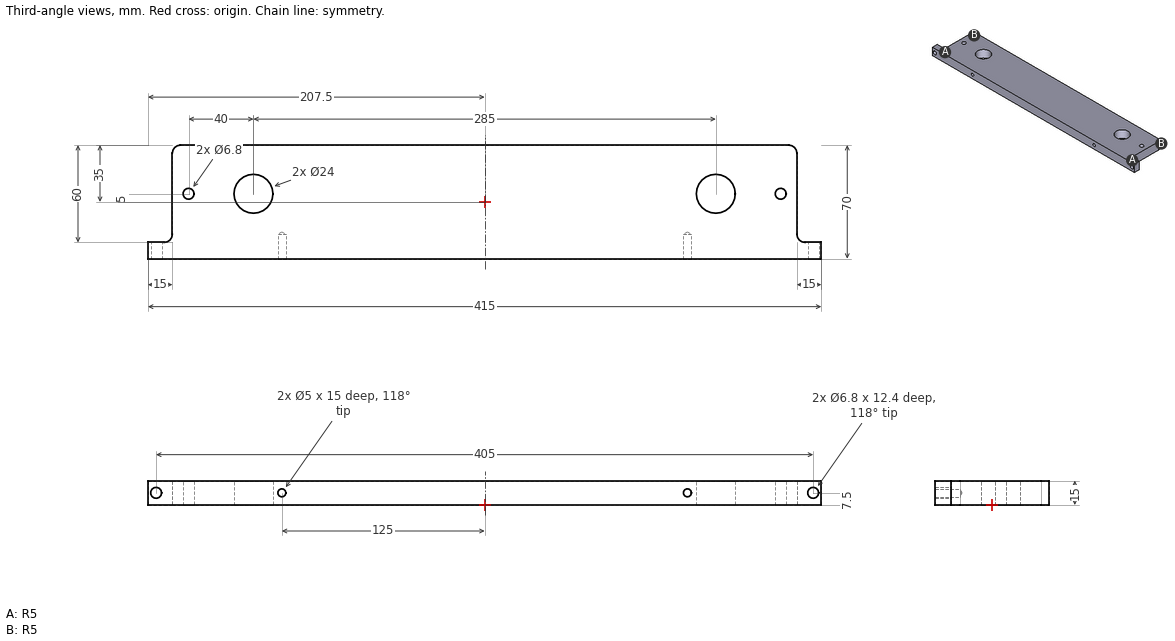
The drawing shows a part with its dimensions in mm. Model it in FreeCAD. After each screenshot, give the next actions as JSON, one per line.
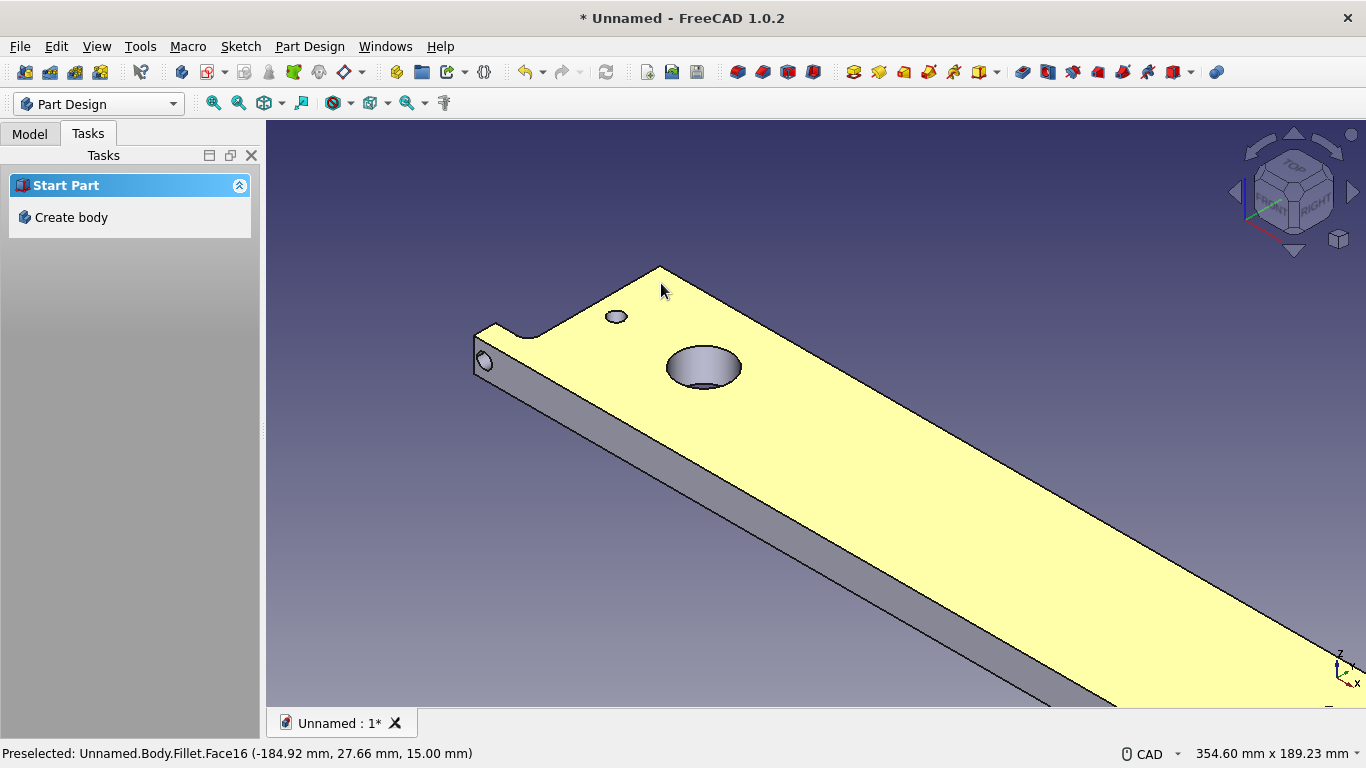
{"action": "key", "text": "v f"}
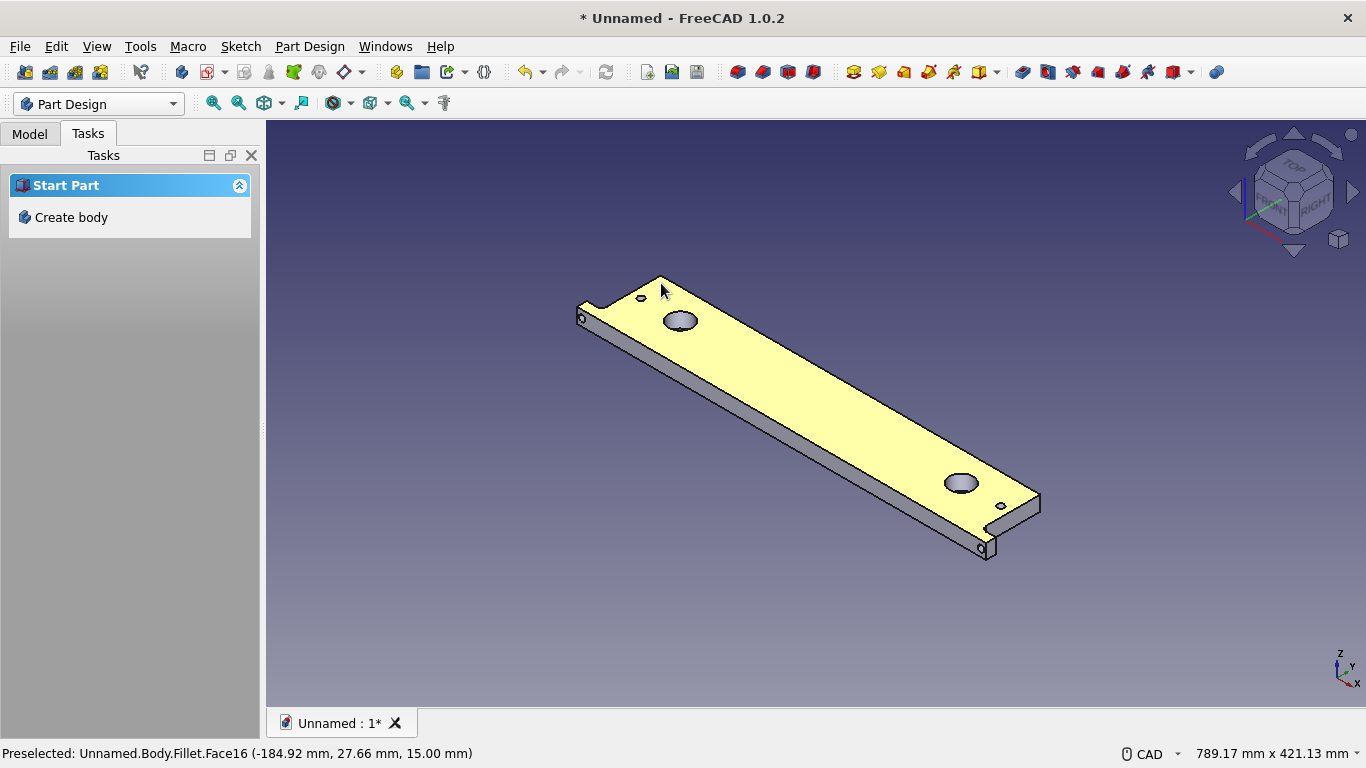
{"action": "key", "text": "2"}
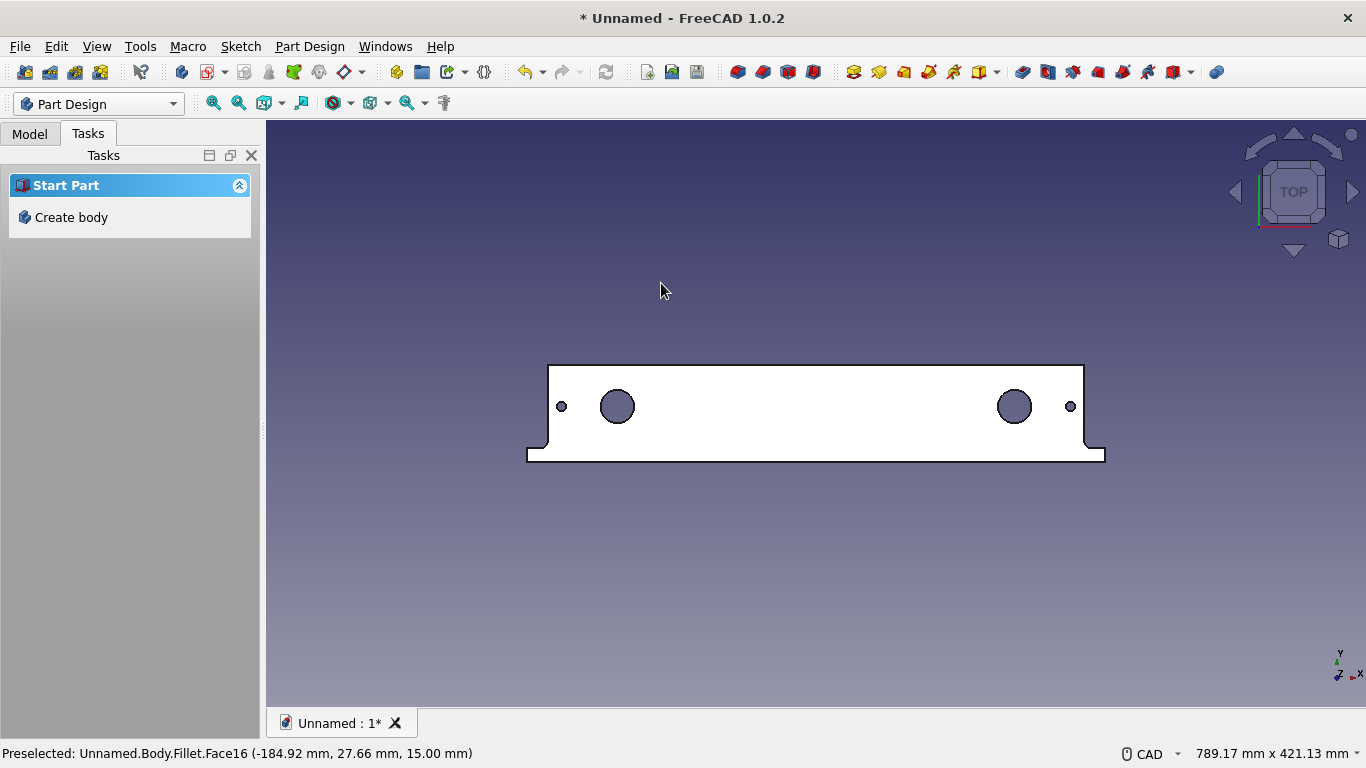
{"action": "scroll", "coordinate": [548, 364], "scroll_direction": "up", "scroll_amount": 4}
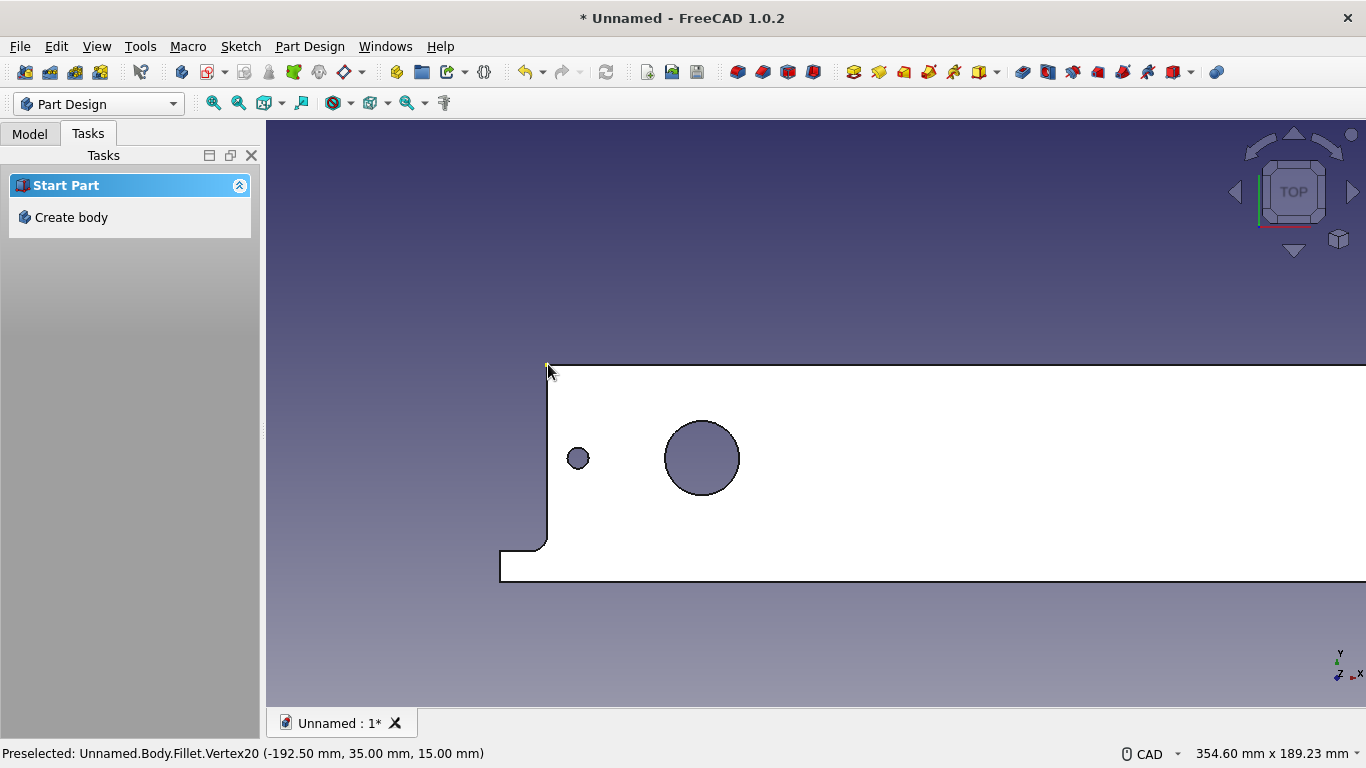
{"action": "left_click", "coordinate": [214, 104]}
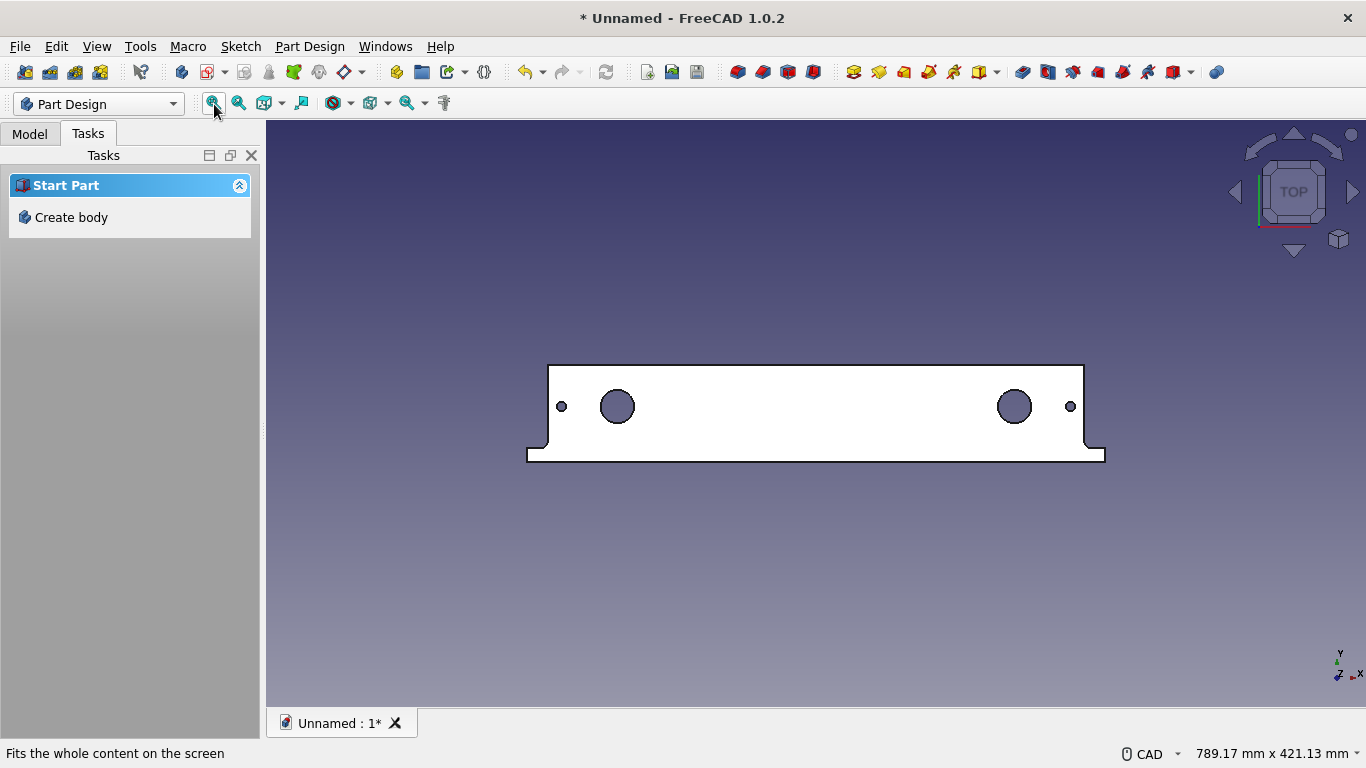
{"action": "key", "text": "1"}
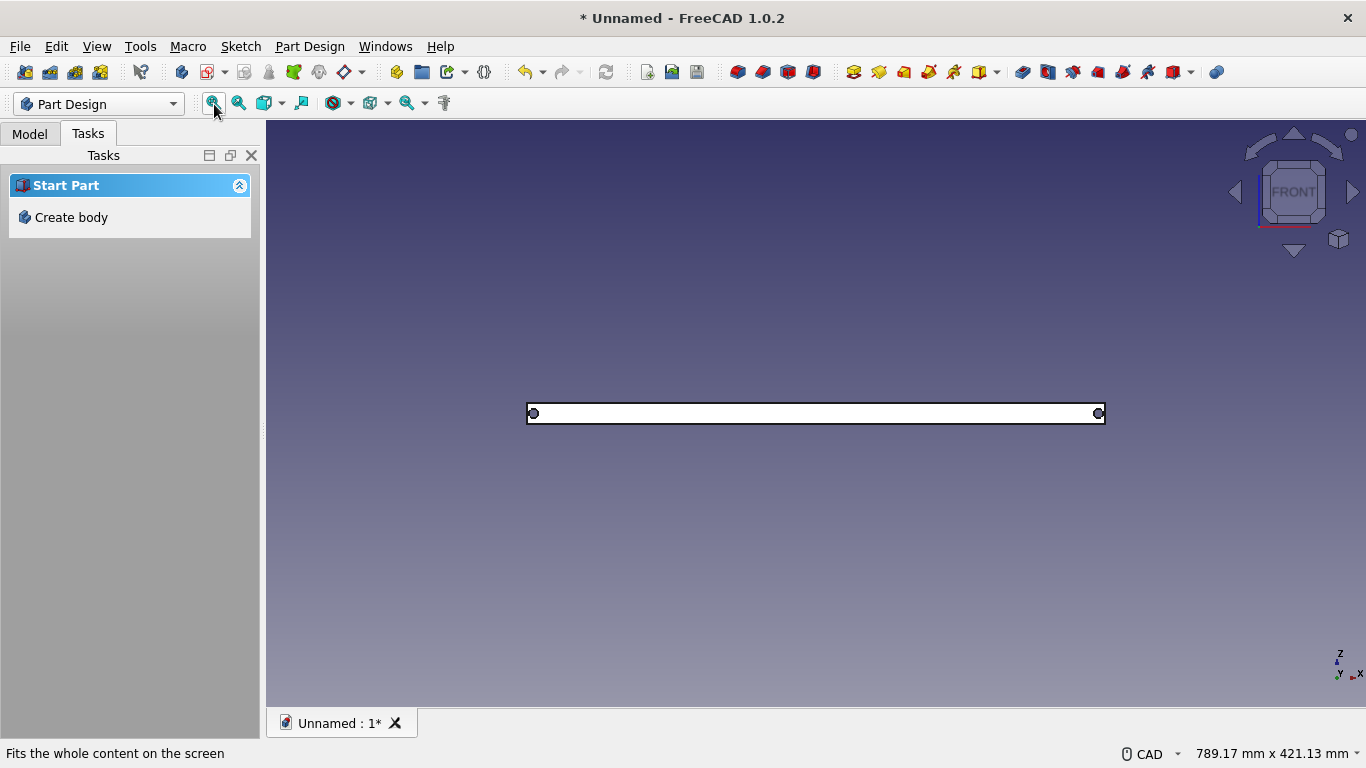
{"action": "scroll", "coordinate": [548, 412], "scroll_direction": "up", "scroll_amount": 4}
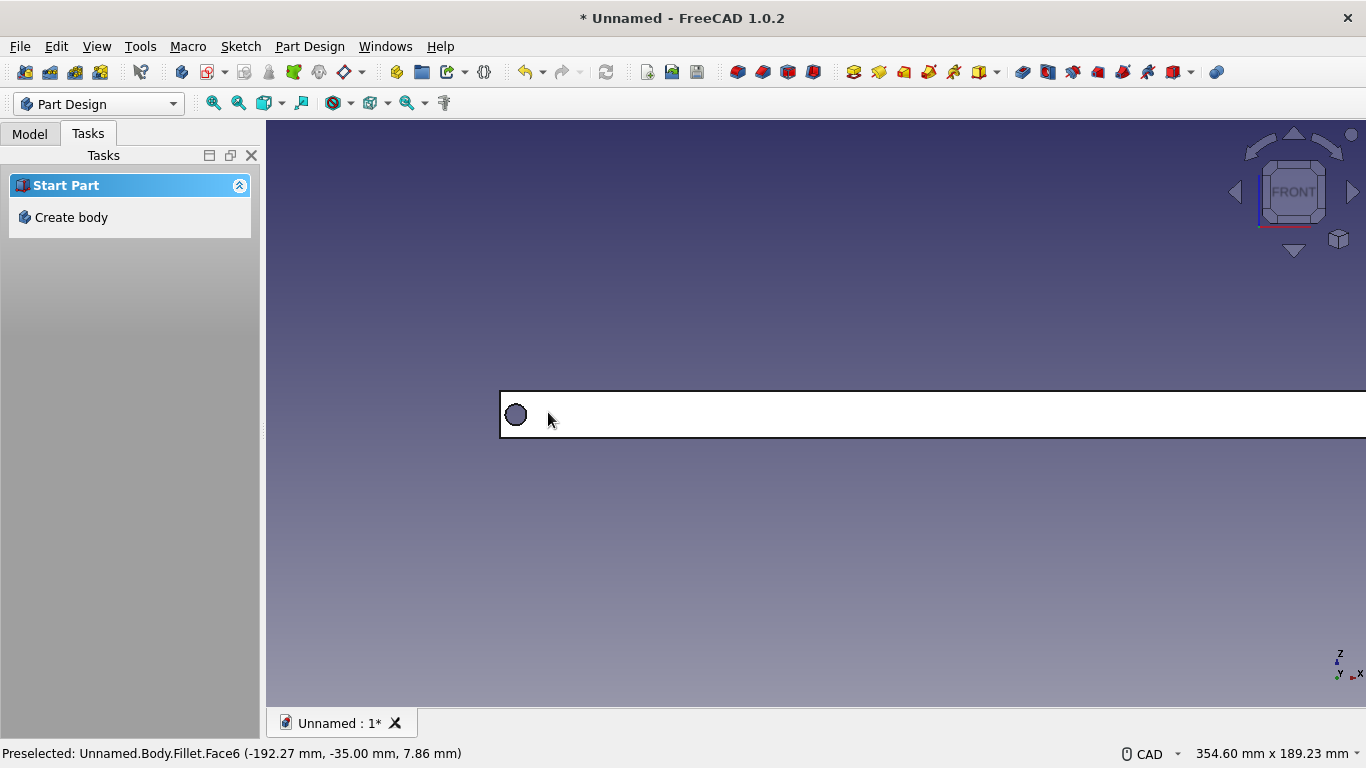
{"action": "key", "text": "v f"}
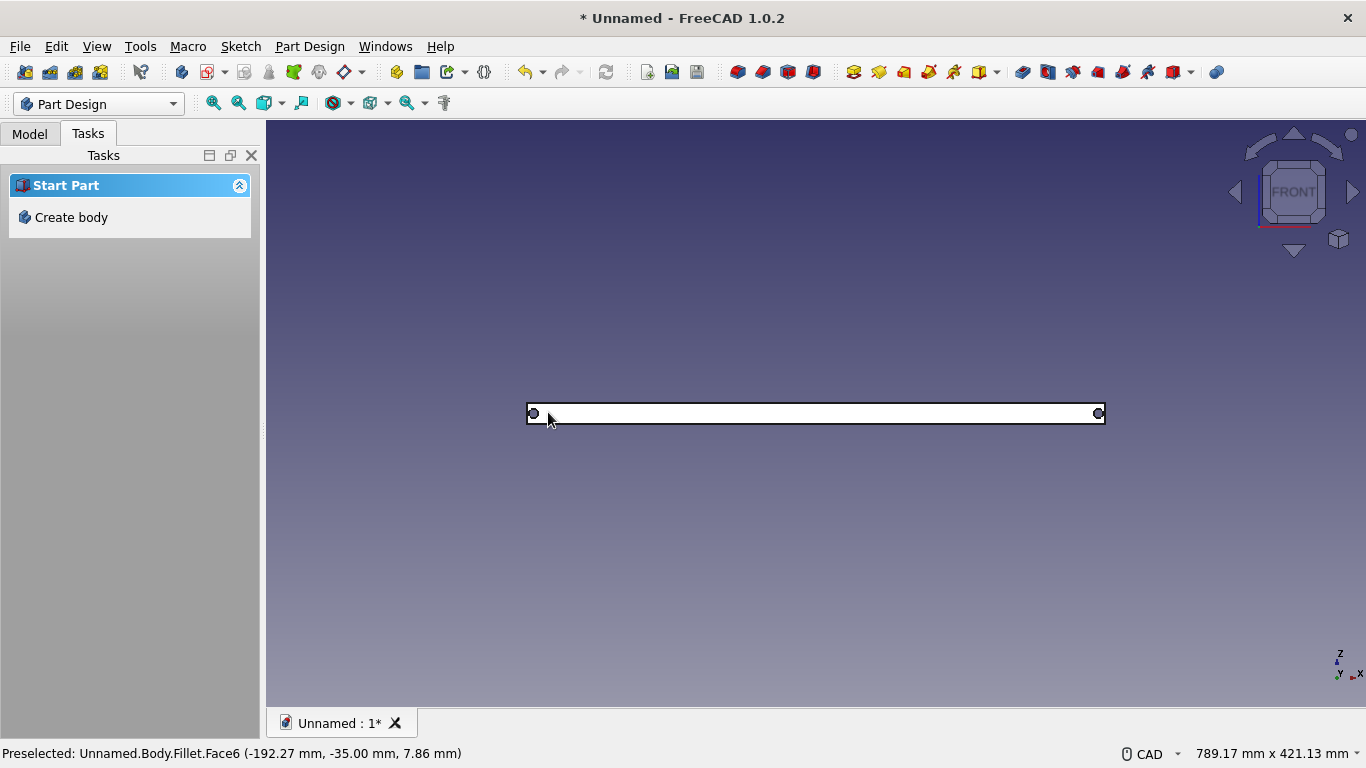
{"action": "key", "text": "3"}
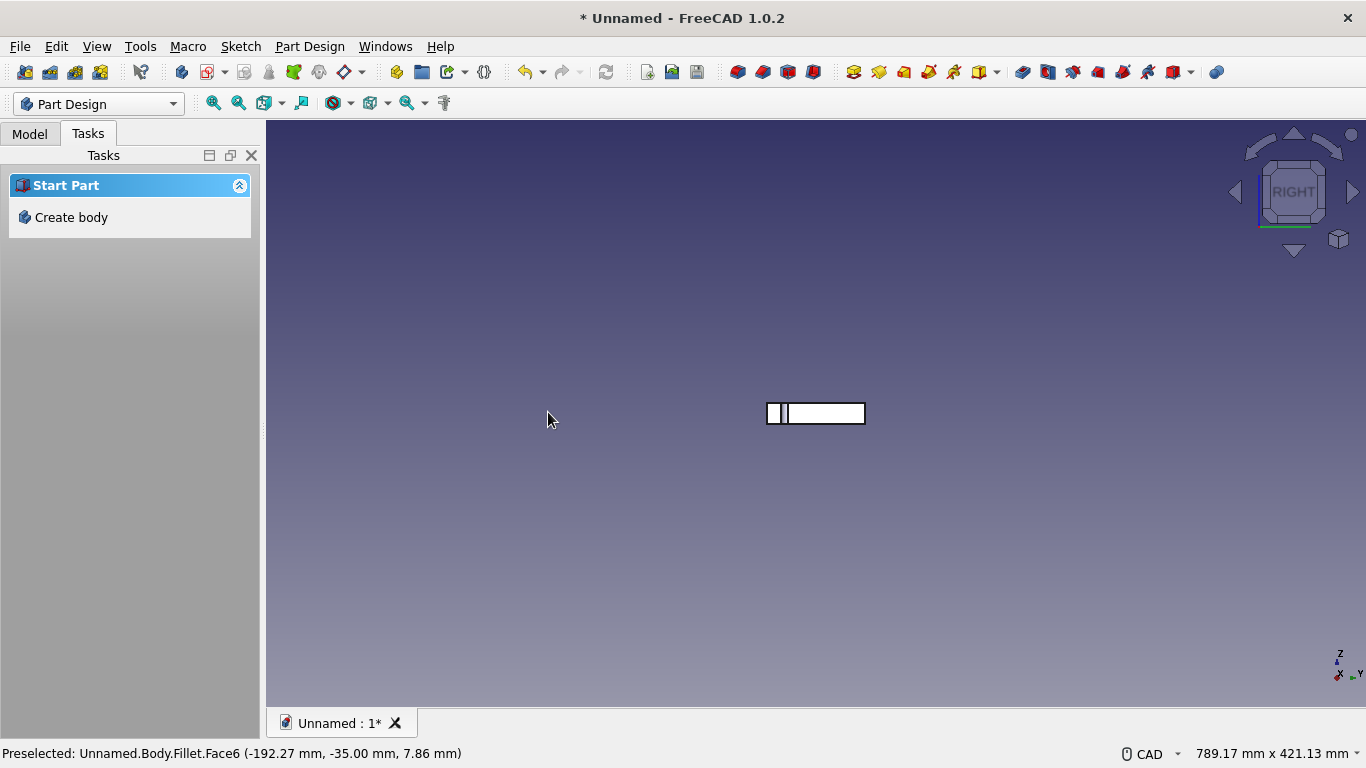
{"action": "key", "text": "v f"}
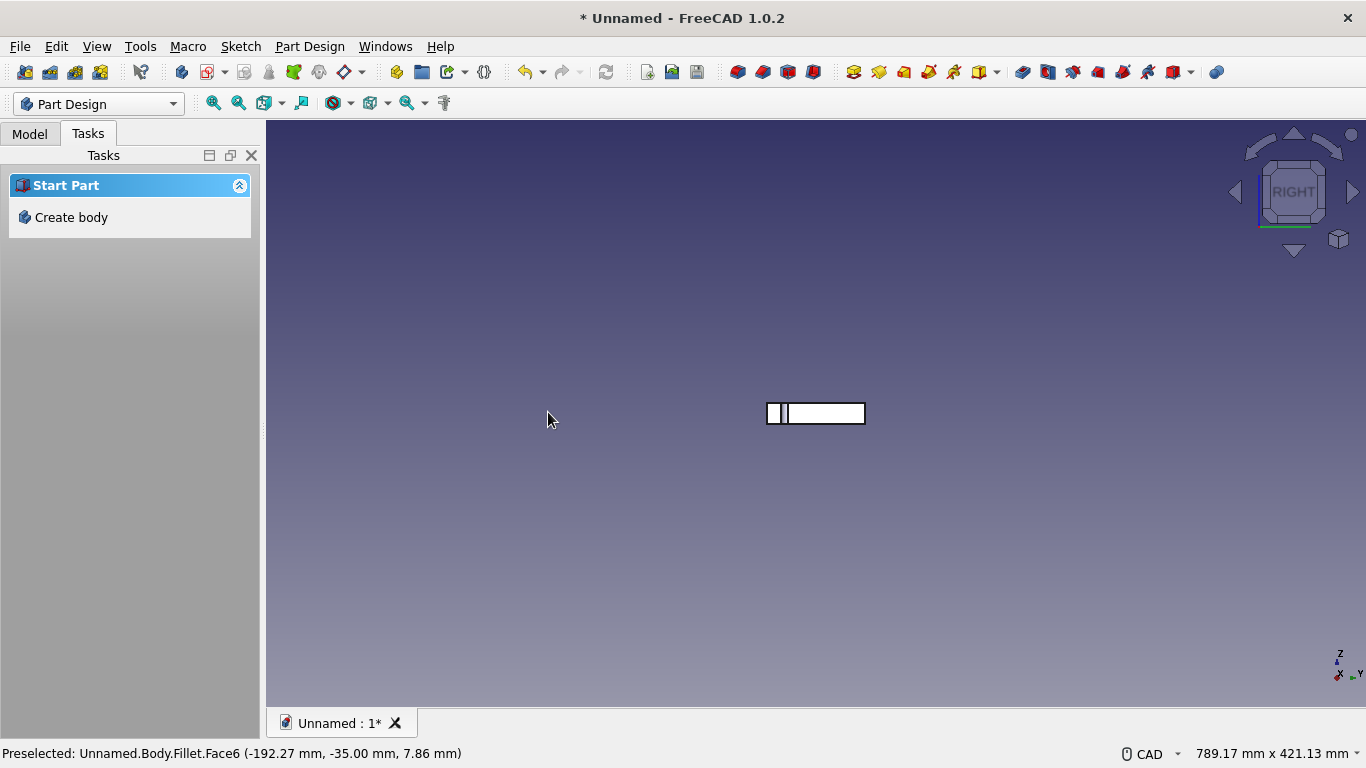
{"action": "left_click", "coordinate": [865, 412]}